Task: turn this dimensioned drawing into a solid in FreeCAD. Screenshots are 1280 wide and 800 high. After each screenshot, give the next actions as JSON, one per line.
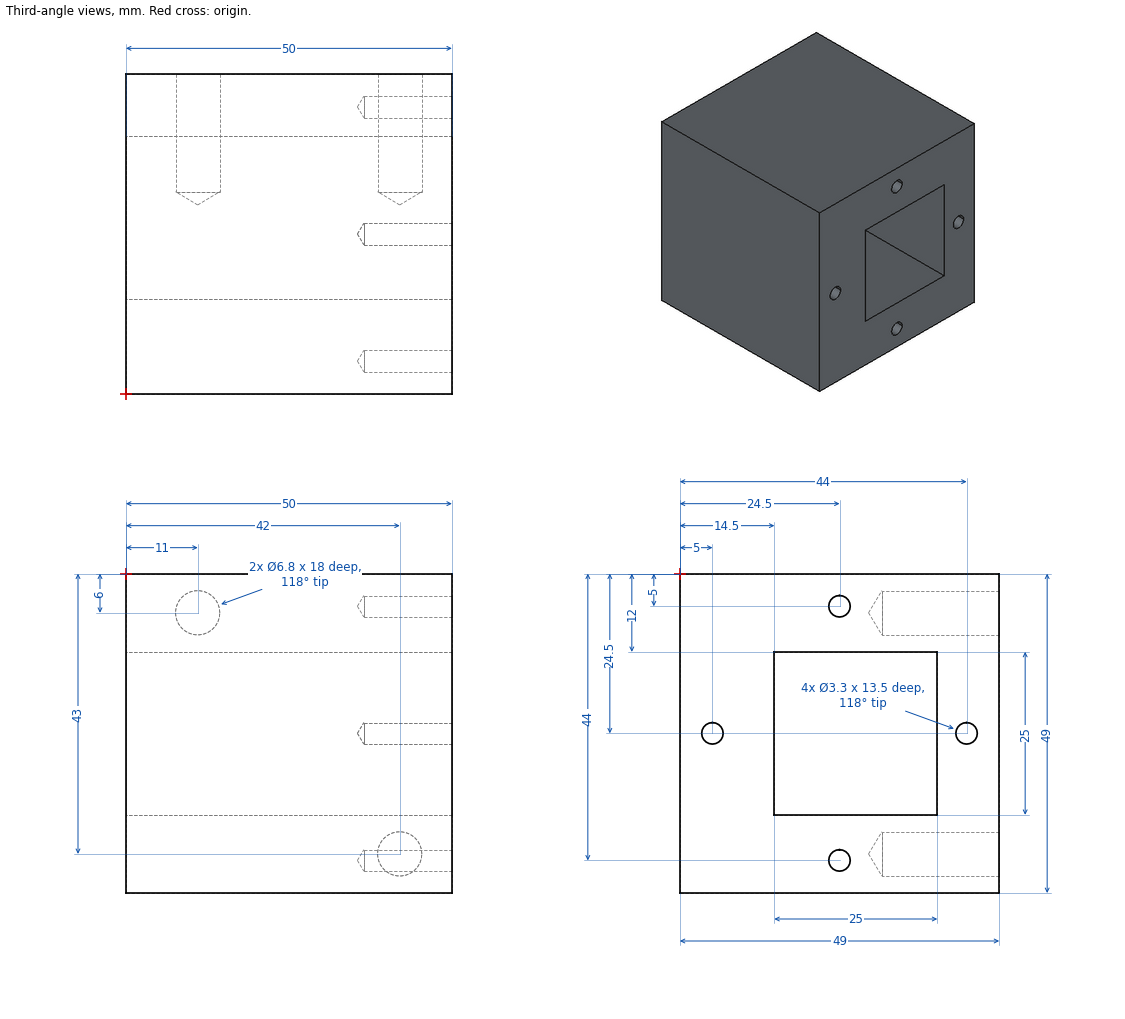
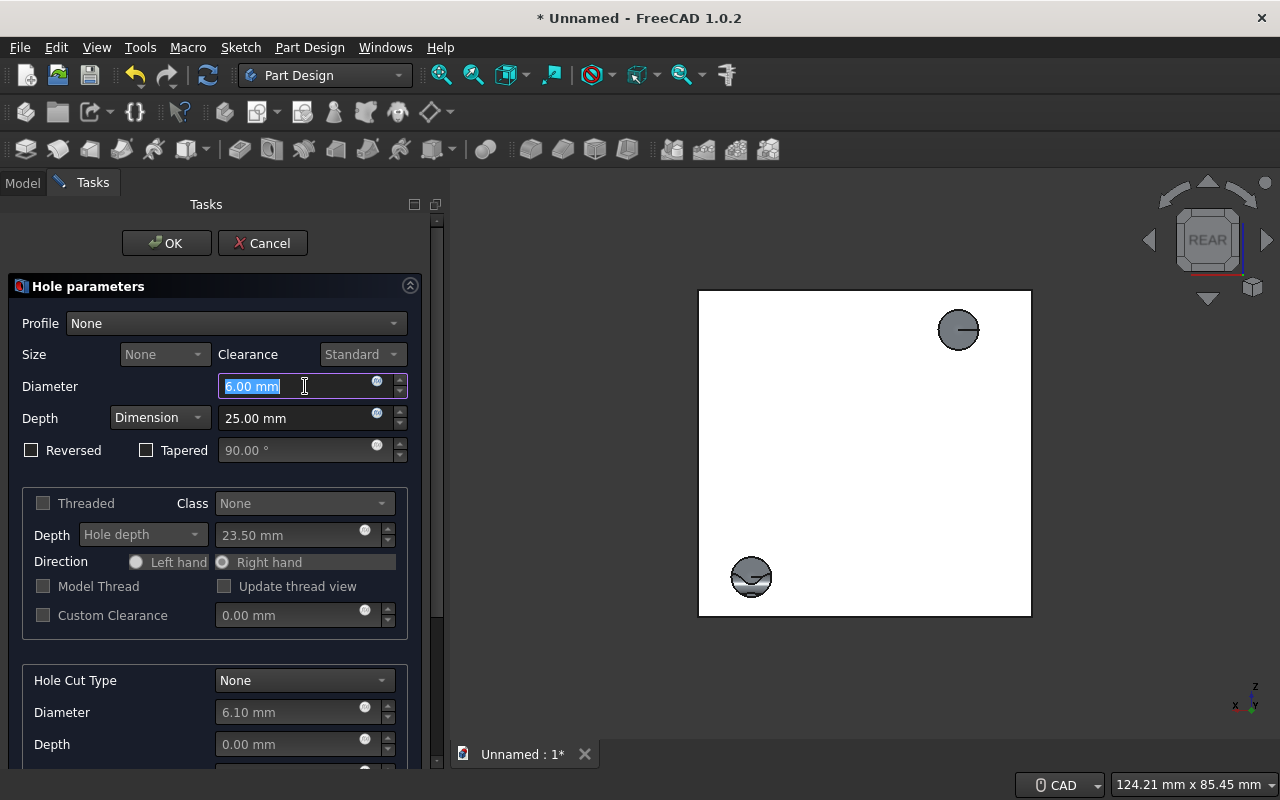
{"action": "type", "text": "6.8"}
{"action": "key", "text": "Tab"}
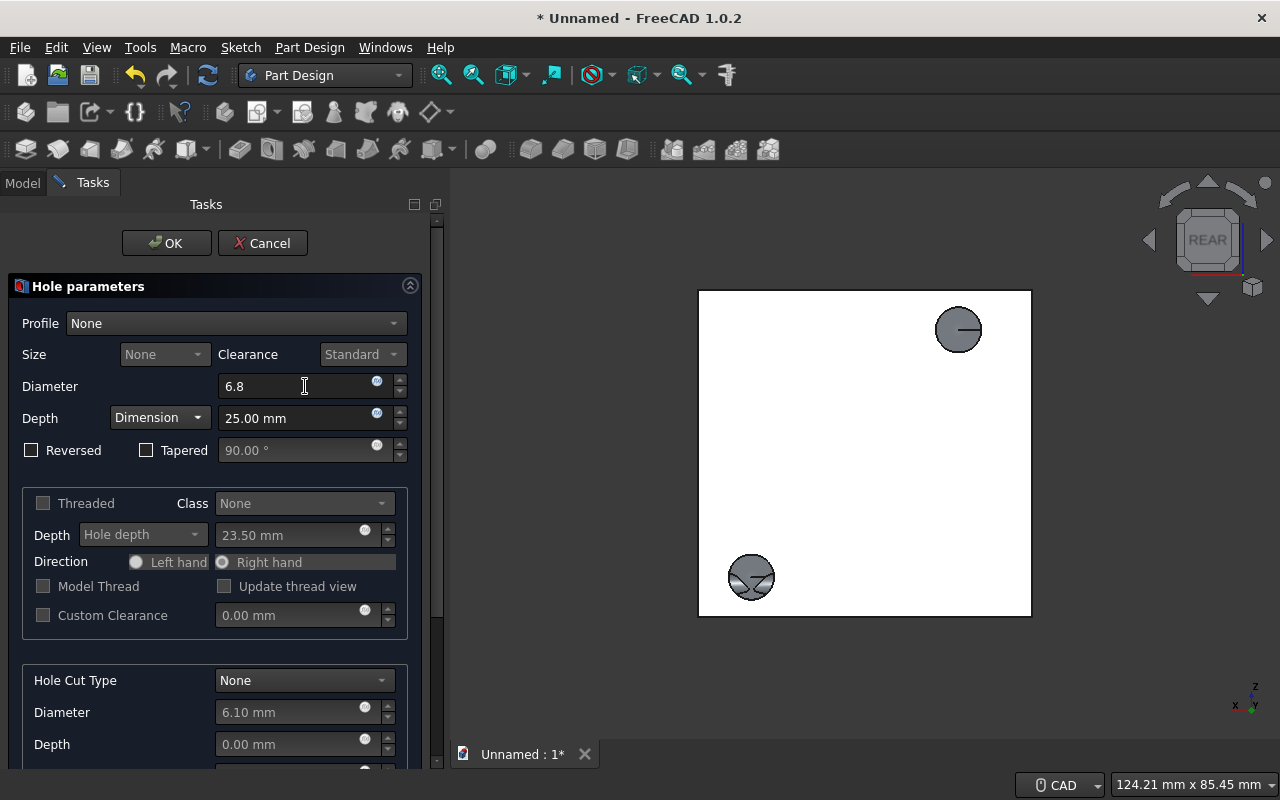
{"action": "triple_click", "coordinate": [305, 418]}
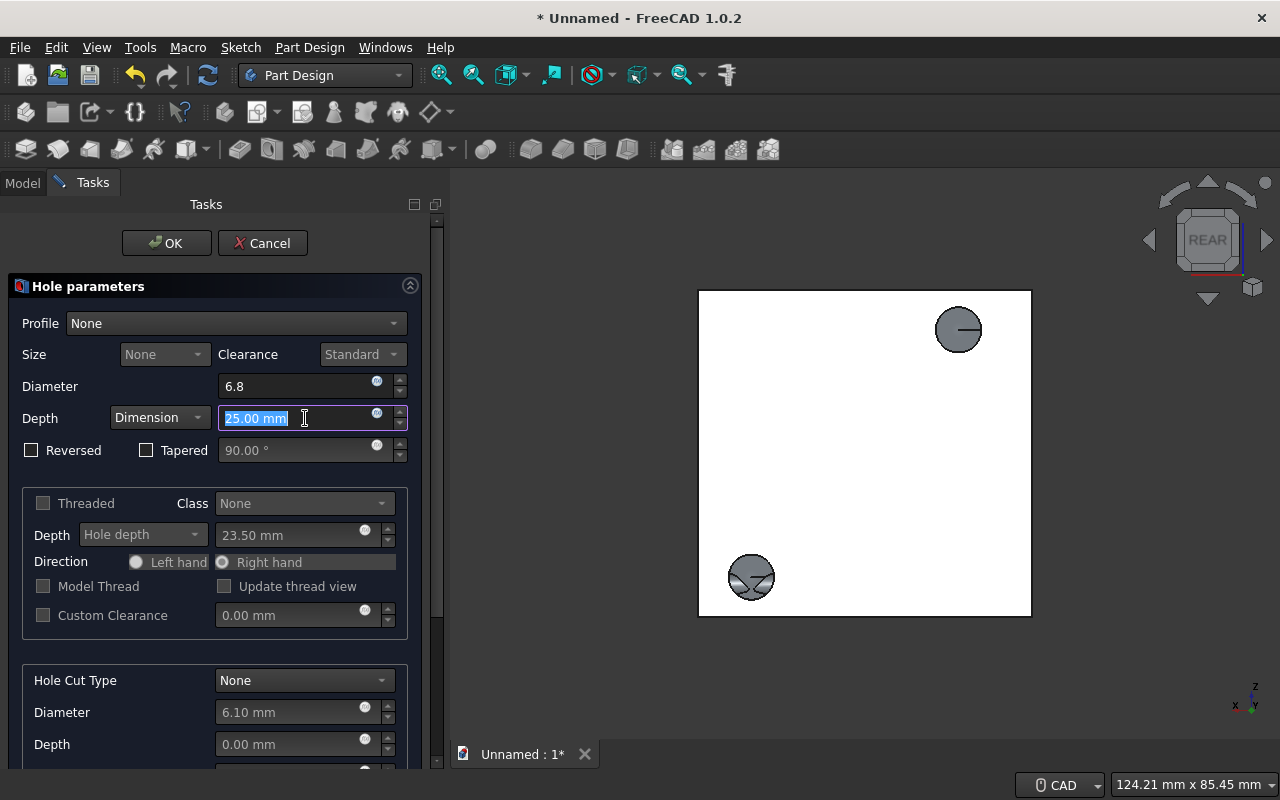
{"action": "type", "text": "18"}
{"action": "key", "text": "Tab"}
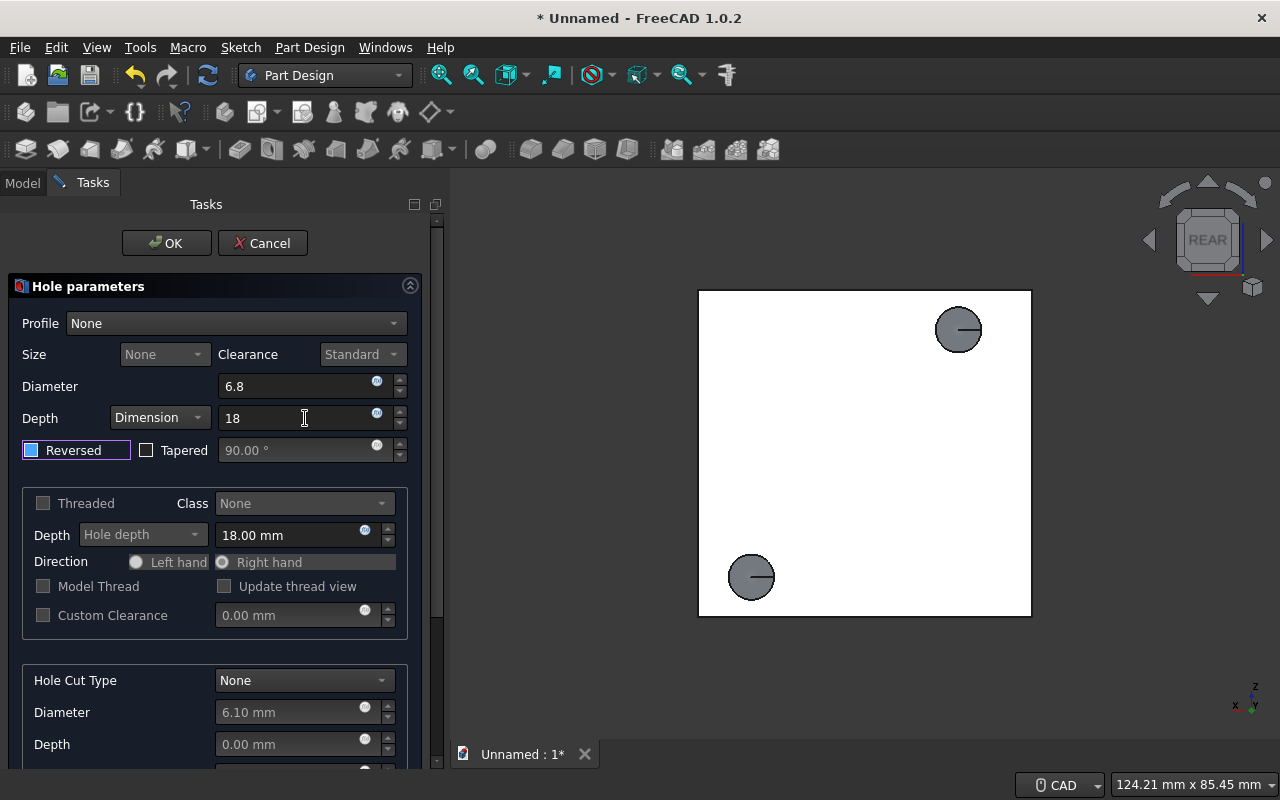
{"action": "left_click", "coordinate": [167, 243]}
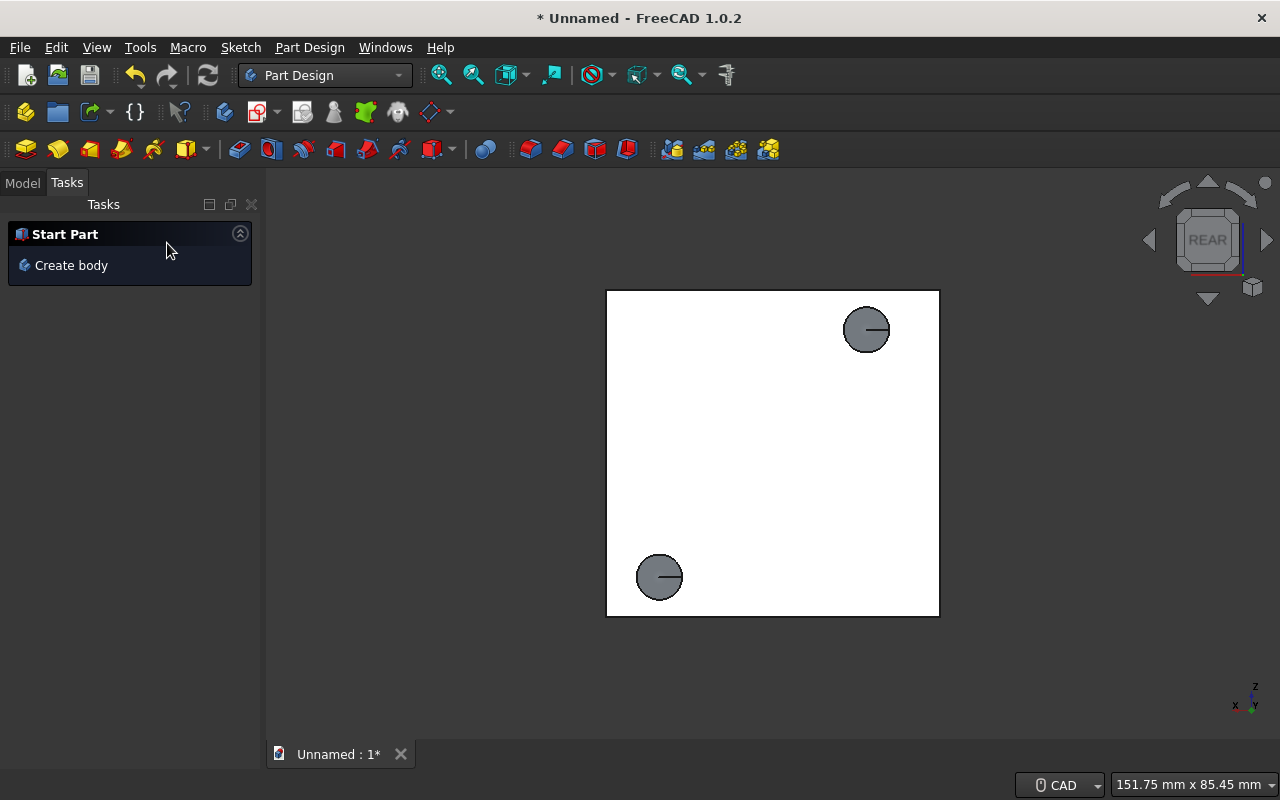
{"action": "key", "text": "0"}